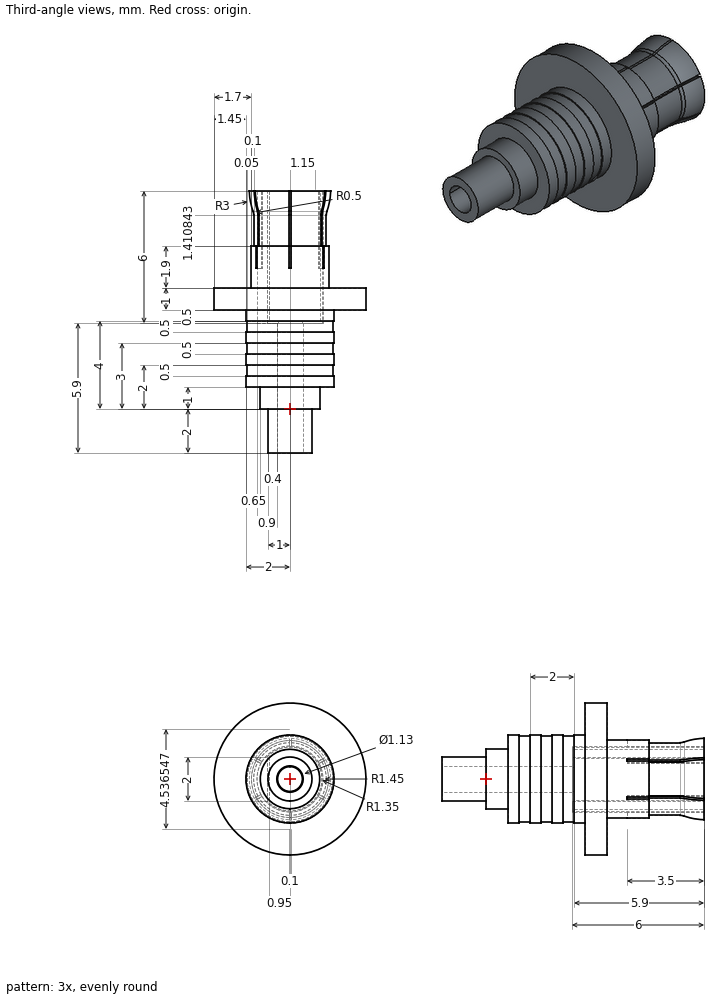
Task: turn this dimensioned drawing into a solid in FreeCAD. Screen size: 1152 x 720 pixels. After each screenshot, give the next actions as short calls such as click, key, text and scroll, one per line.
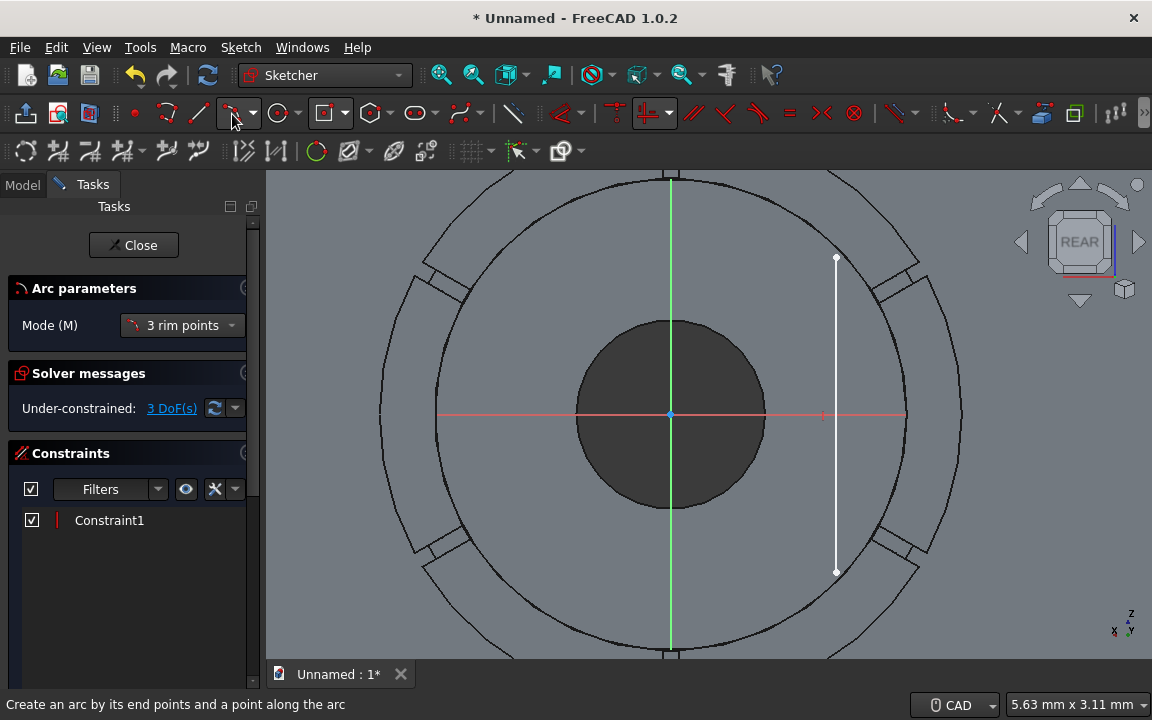
click(836, 258)
click(836, 573)
click(468, 310)
key(Escape)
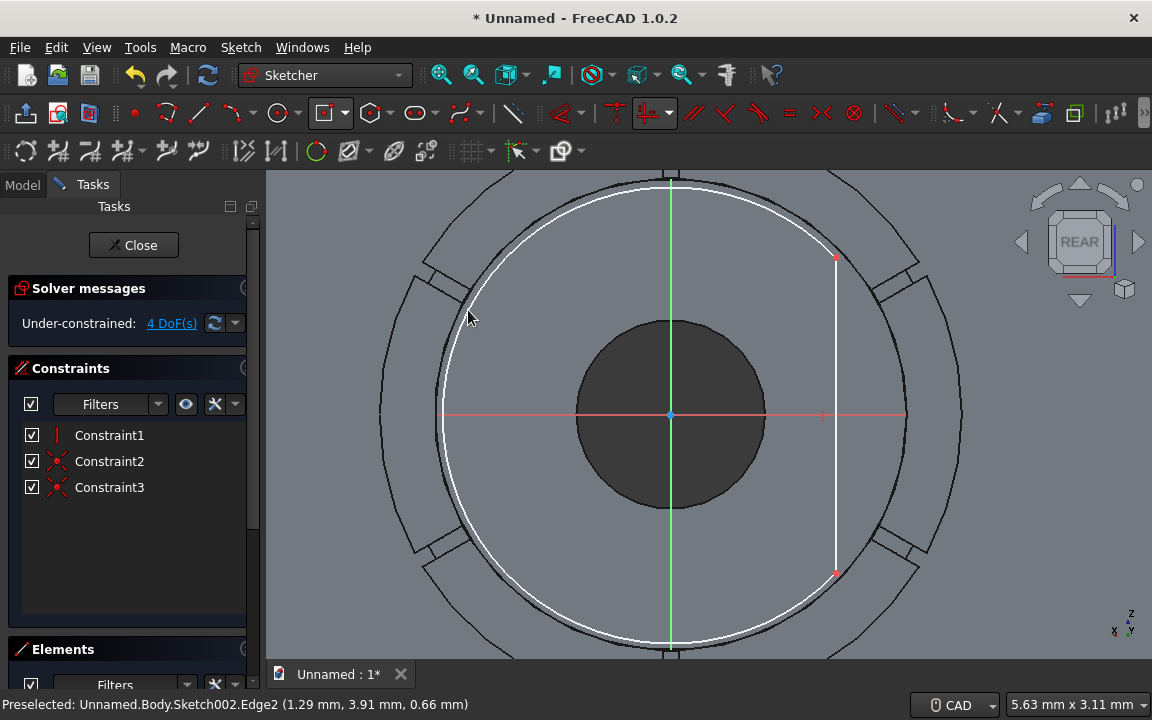
drag(661, 404, 681, 426)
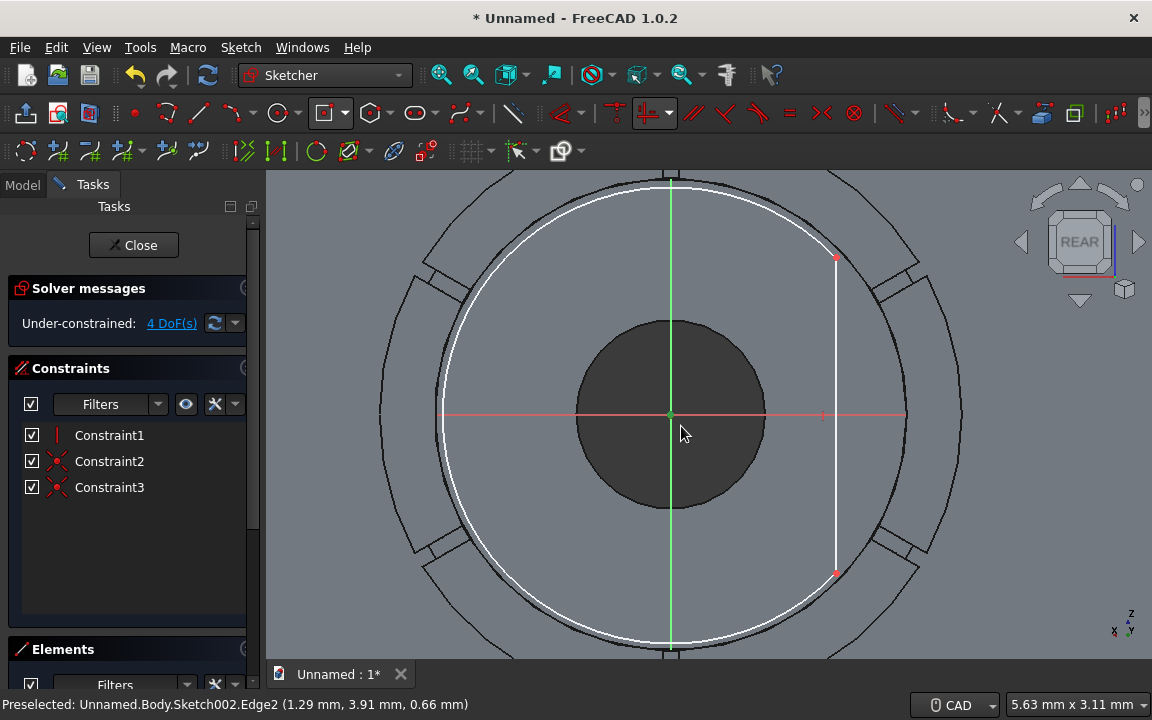
click(616, 114)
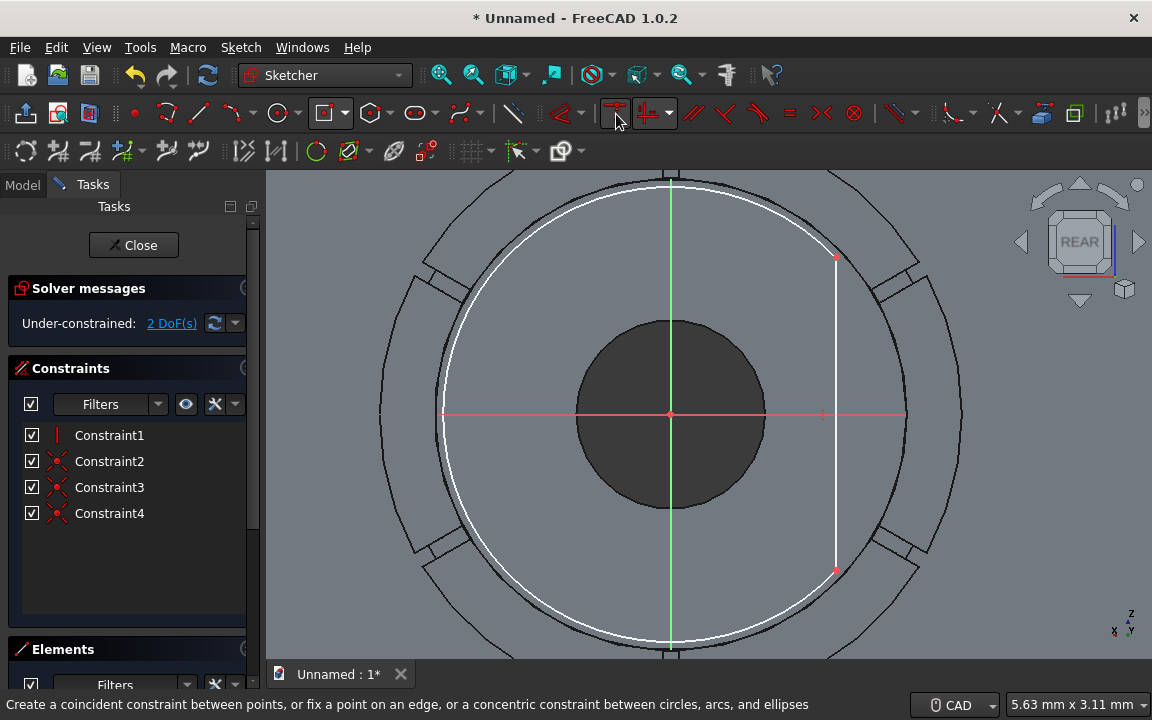
click(560, 114)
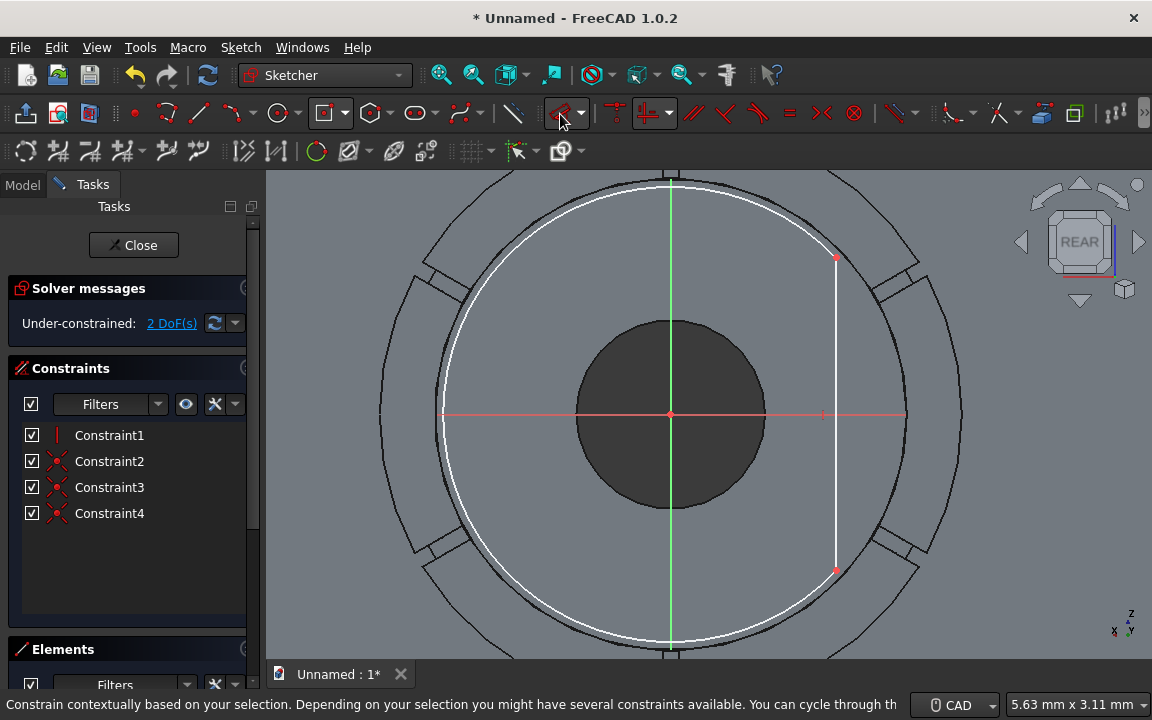
click(539, 229)
click(520, 203)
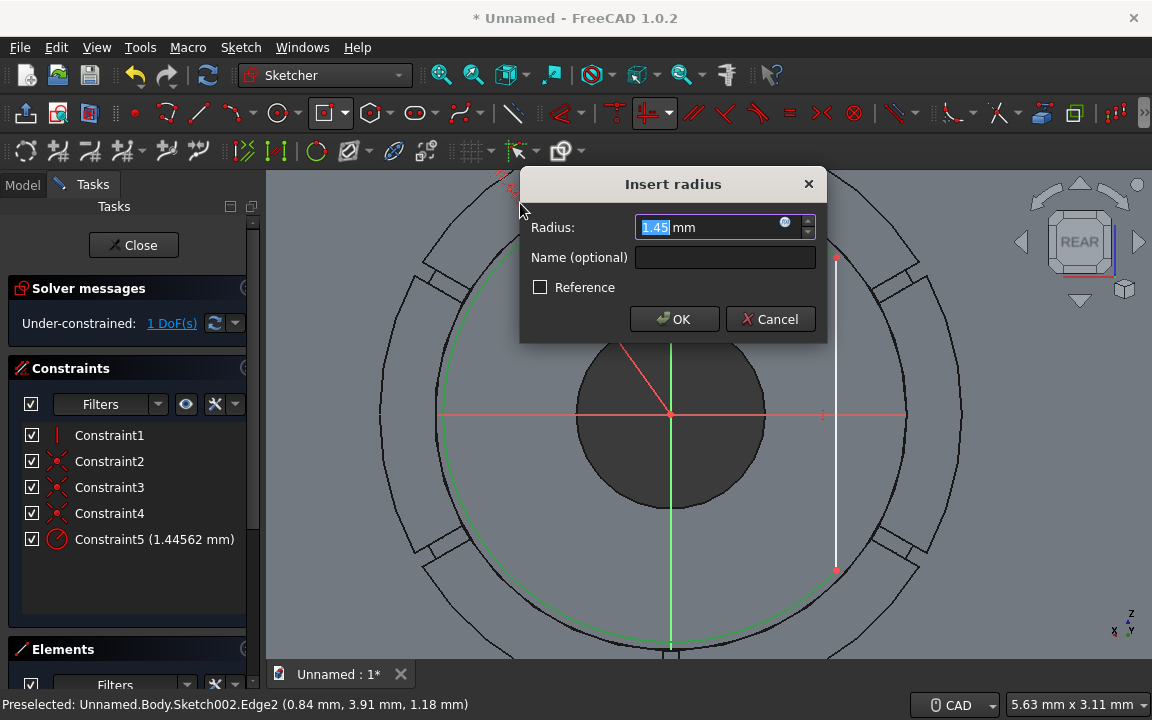
text(1.45)
key(Return)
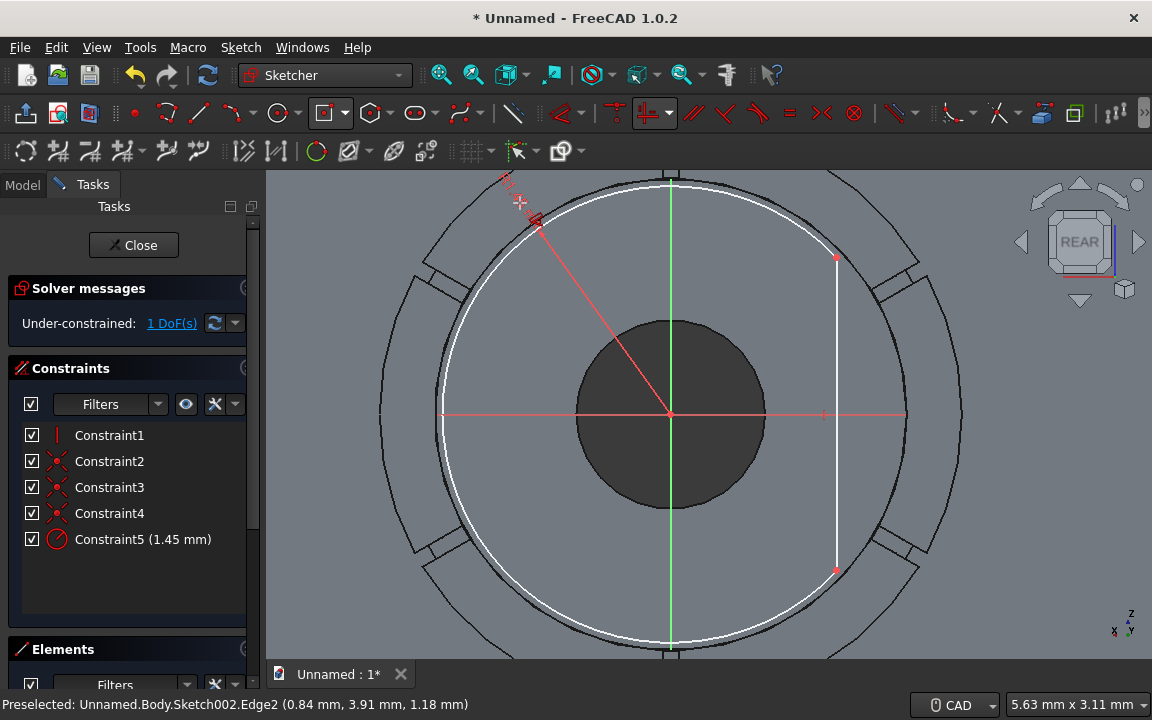
click(837, 477)
click(871, 343)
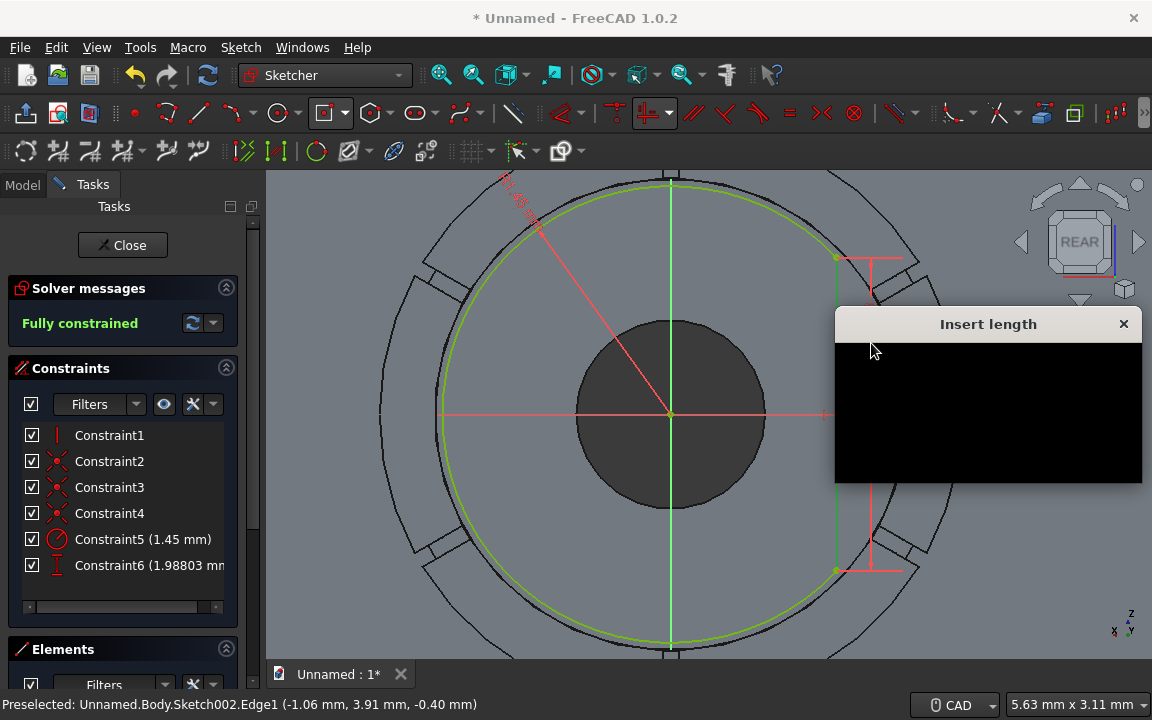
text(2)
key(Return)
key(Escape)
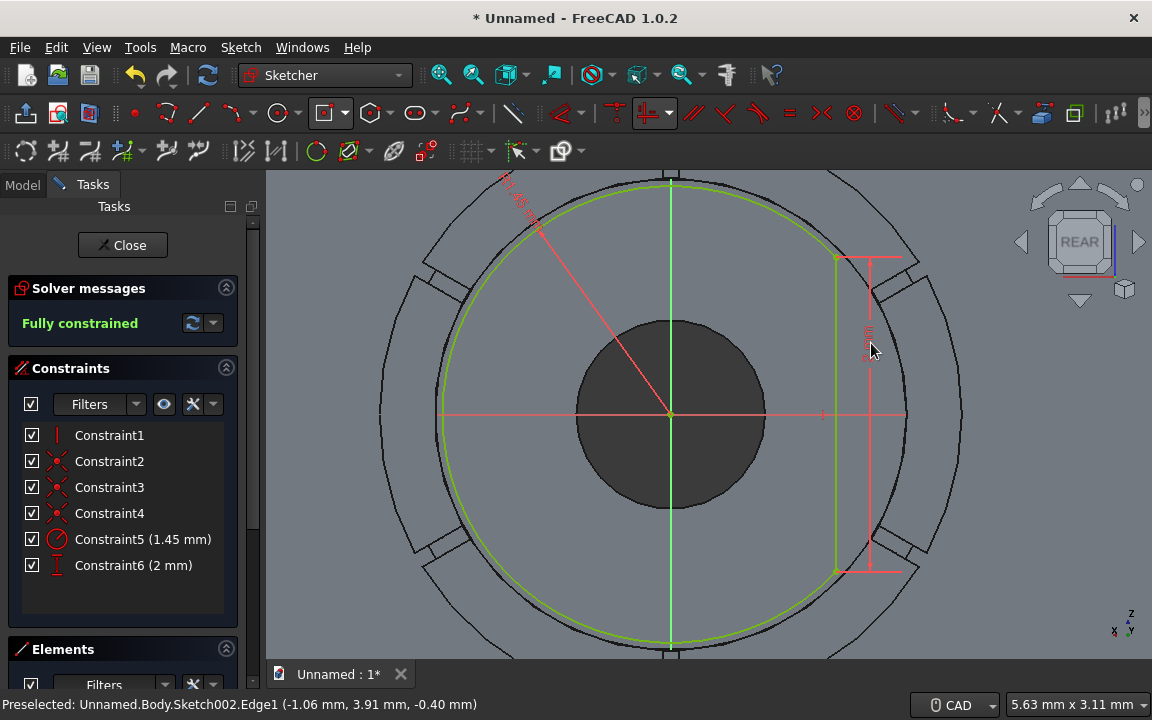
click(123, 245)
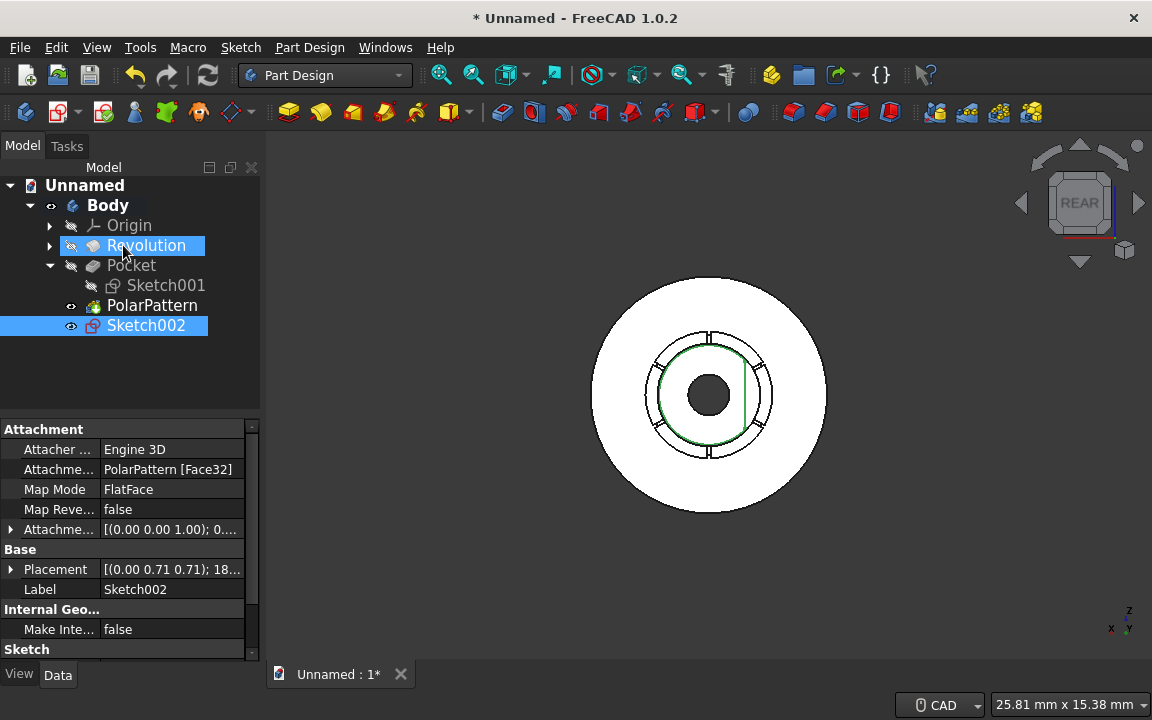
click(290, 112)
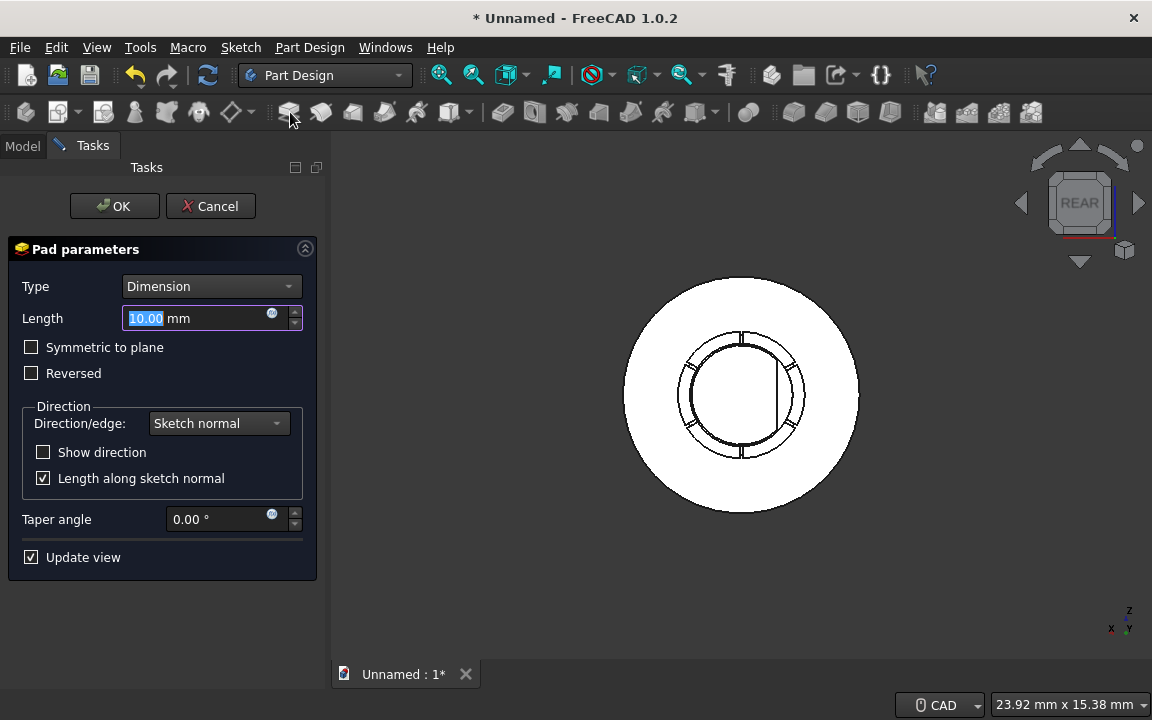
text(6)
key(Tab)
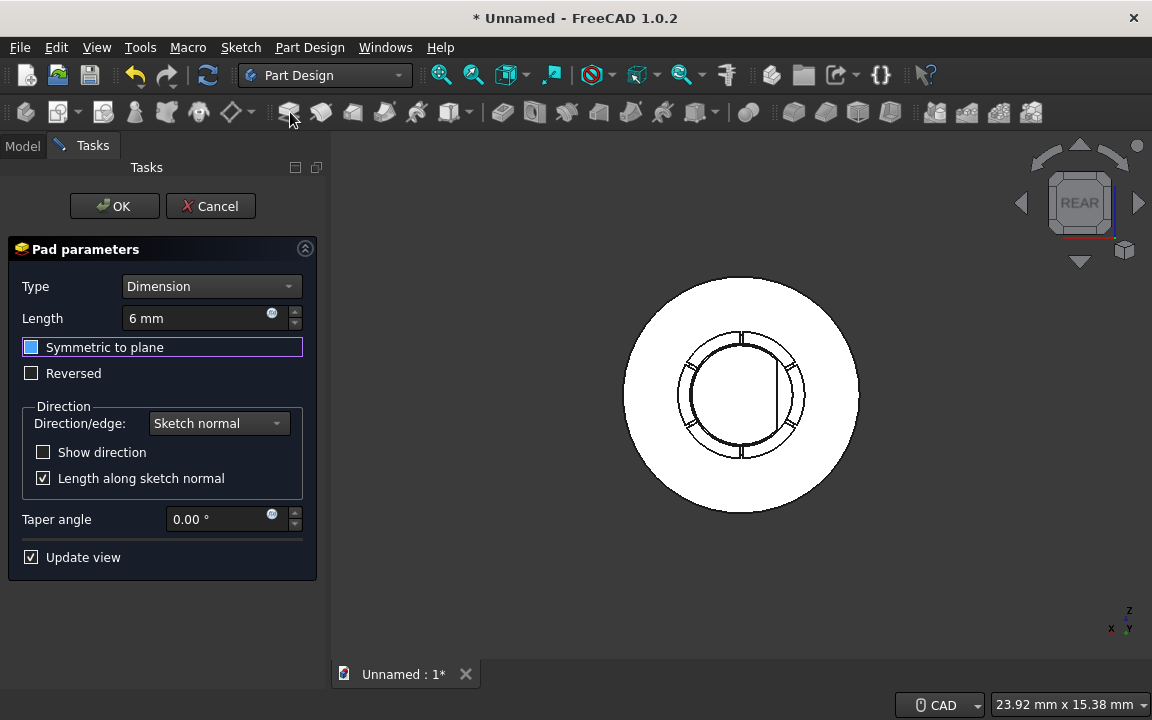
click(115, 206)